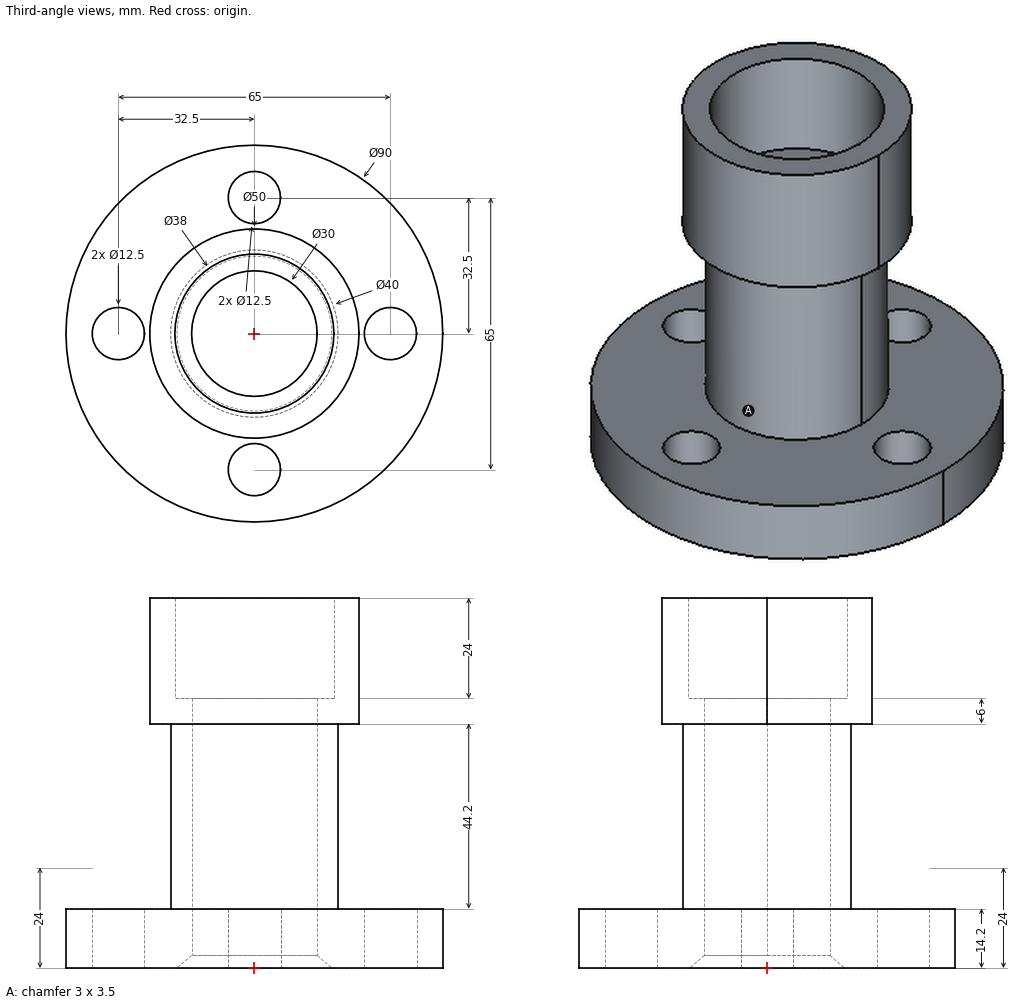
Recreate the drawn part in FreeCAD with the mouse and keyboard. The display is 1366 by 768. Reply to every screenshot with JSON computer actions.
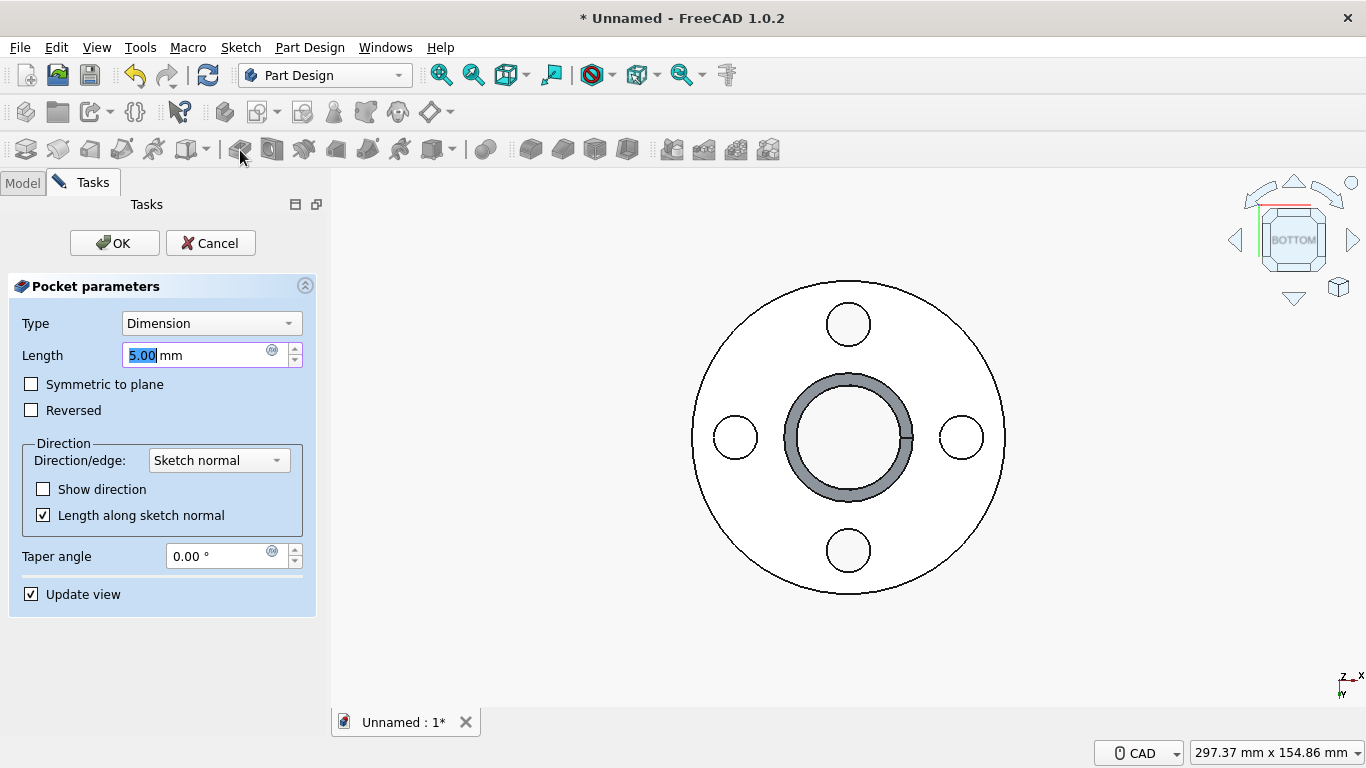
{"action": "type", "text": "24"}
{"action": "key", "text": "Tab"}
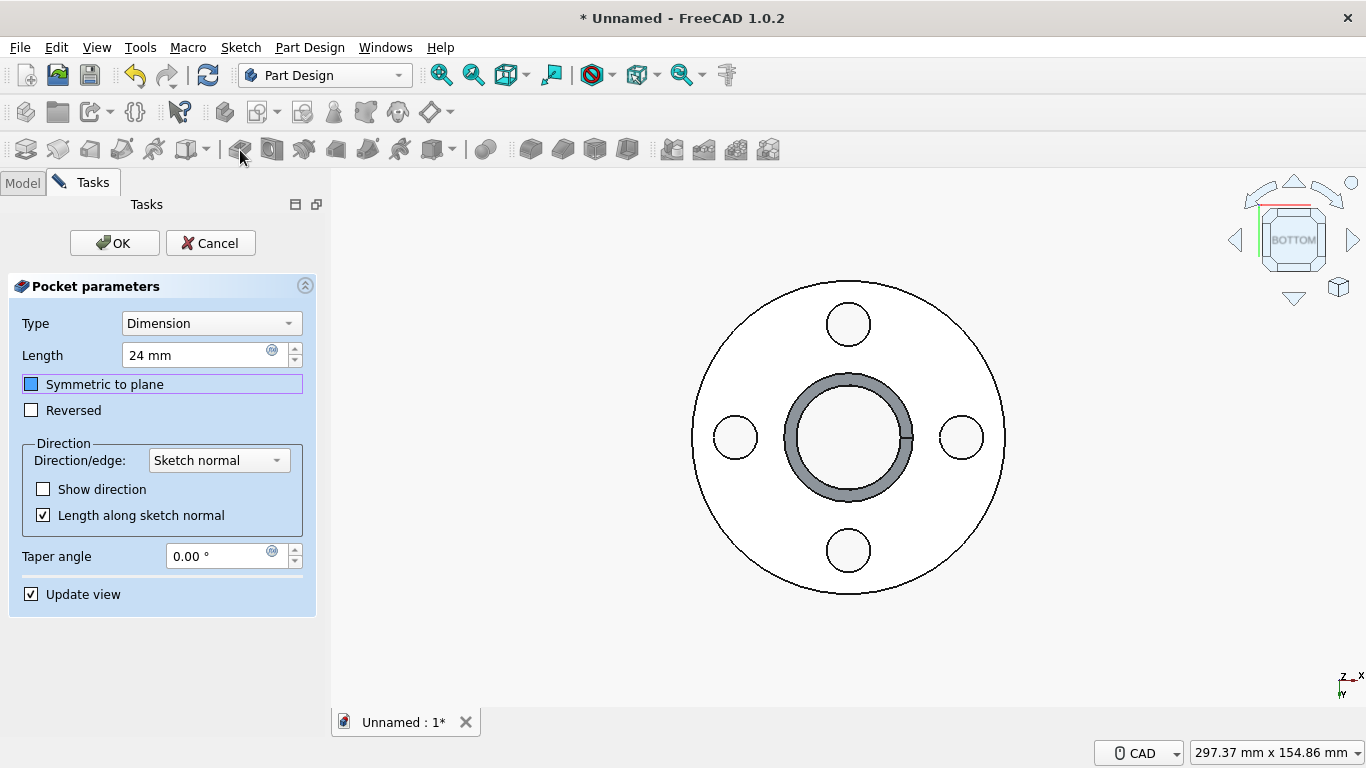
{"action": "left_click", "coordinate": [115, 243]}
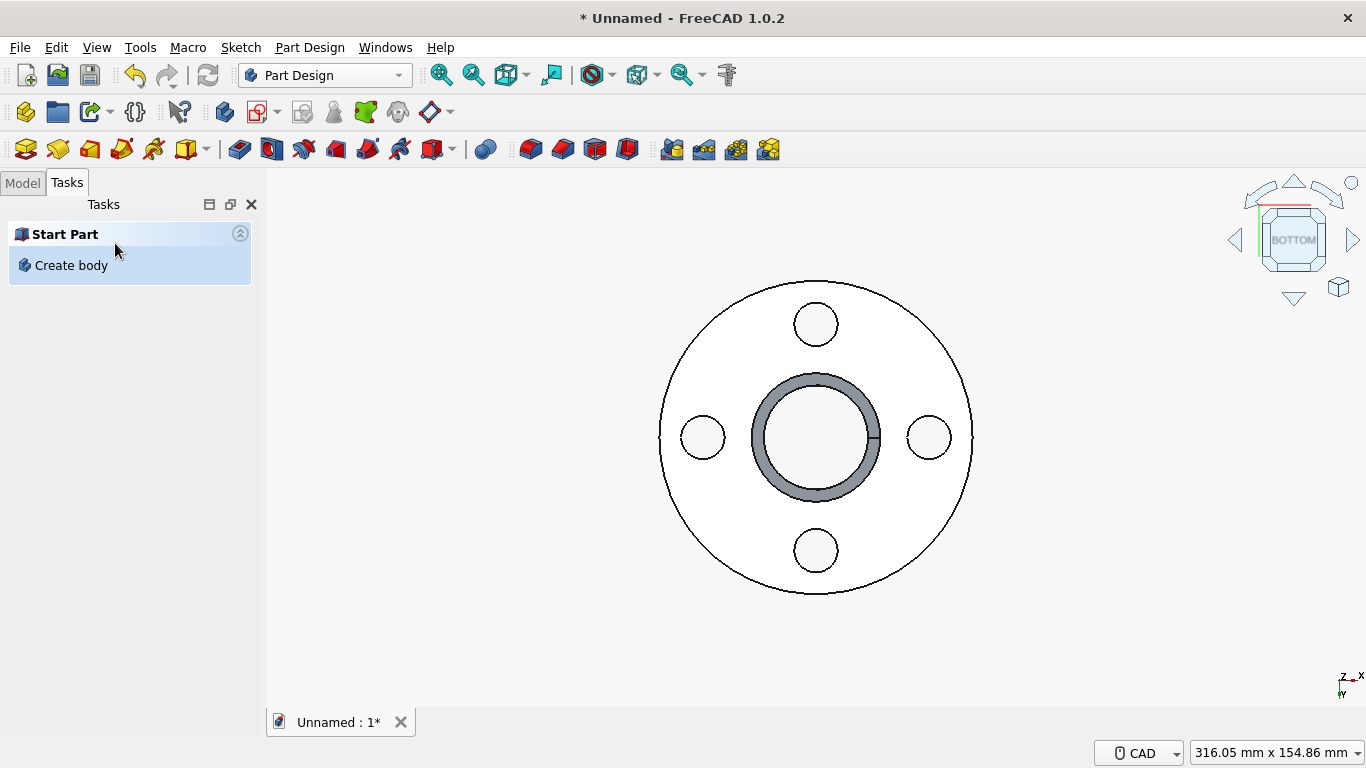
{"action": "key", "text": "0"}